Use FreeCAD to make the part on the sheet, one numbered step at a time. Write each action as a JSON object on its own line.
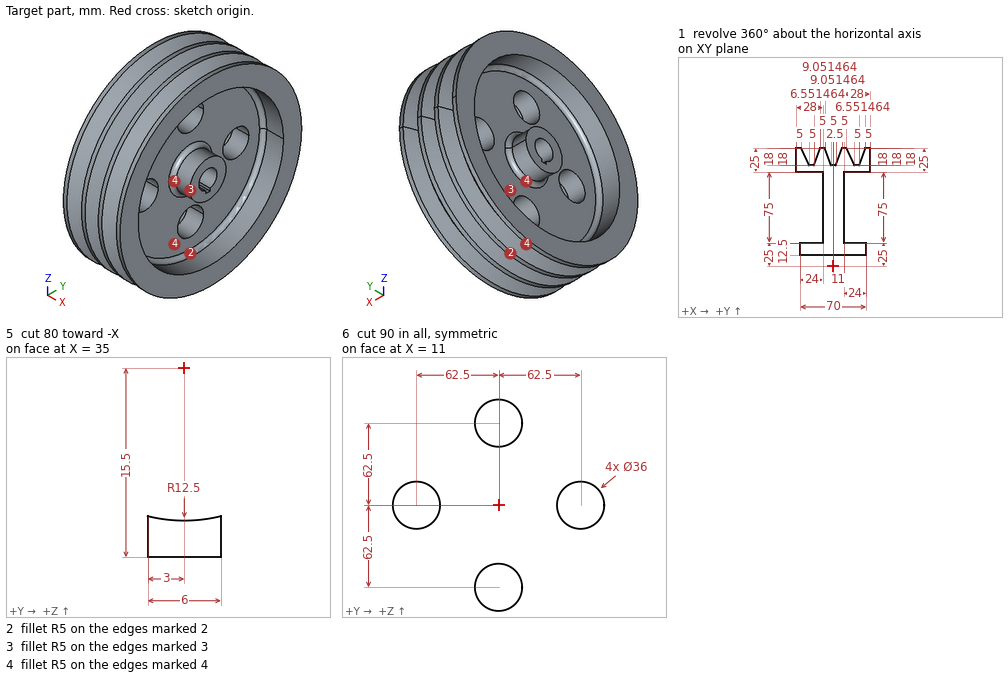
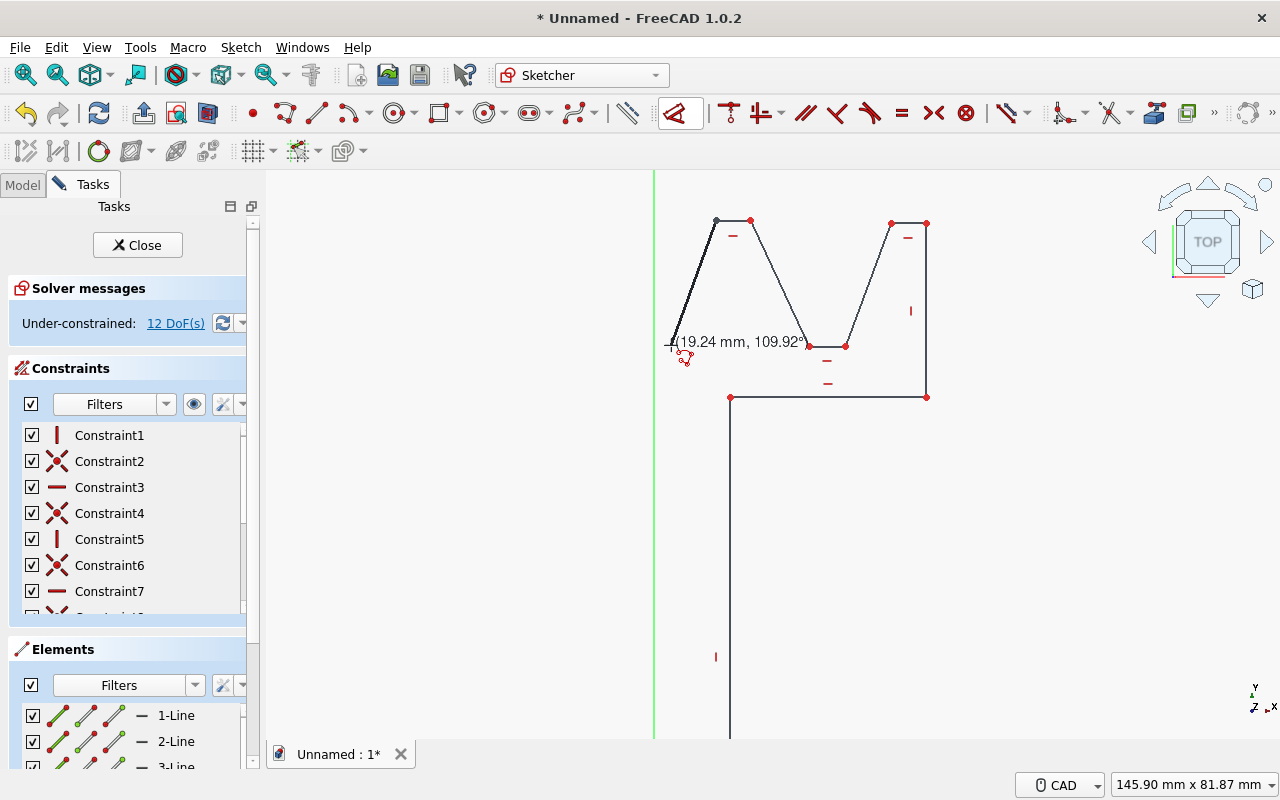
{"action": "left_click", "coordinate": [671, 345]}
{"action": "left_click", "coordinate": [637, 345]}
{"action": "left_click", "coordinate": [591, 220]}
{"action": "left_click", "coordinate": [556, 220]}
{"action": "left_click", "coordinate": [511, 345]}
{"action": "left_click", "coordinate": [476, 345]}
{"action": "left_click", "coordinate": [418, 220]}
{"action": "left_click", "coordinate": [383, 220]}
{"action": "left_click", "coordinate": [383, 394]}
{"action": "left_click", "coordinate": [578, 394]}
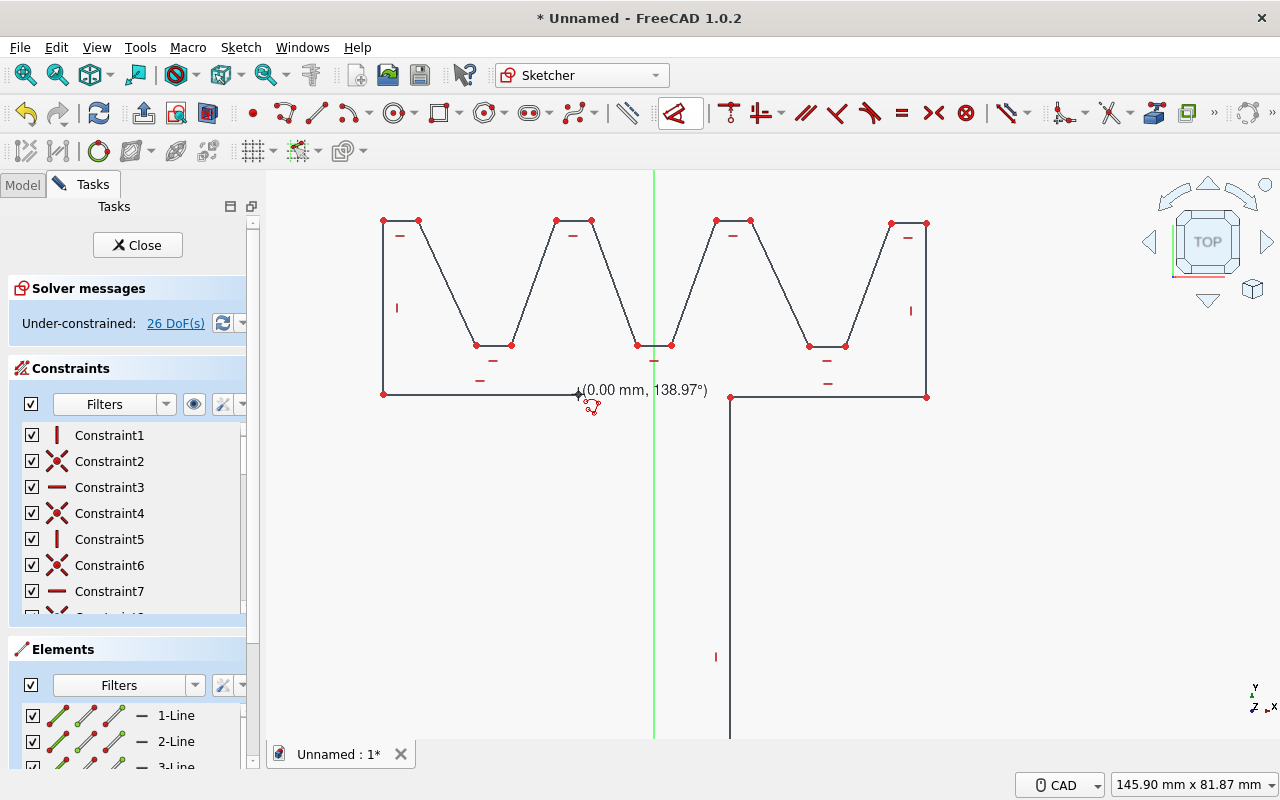
{"action": "scroll", "coordinate": [746, 292], "scroll_direction": "down", "scroll_amount": 4}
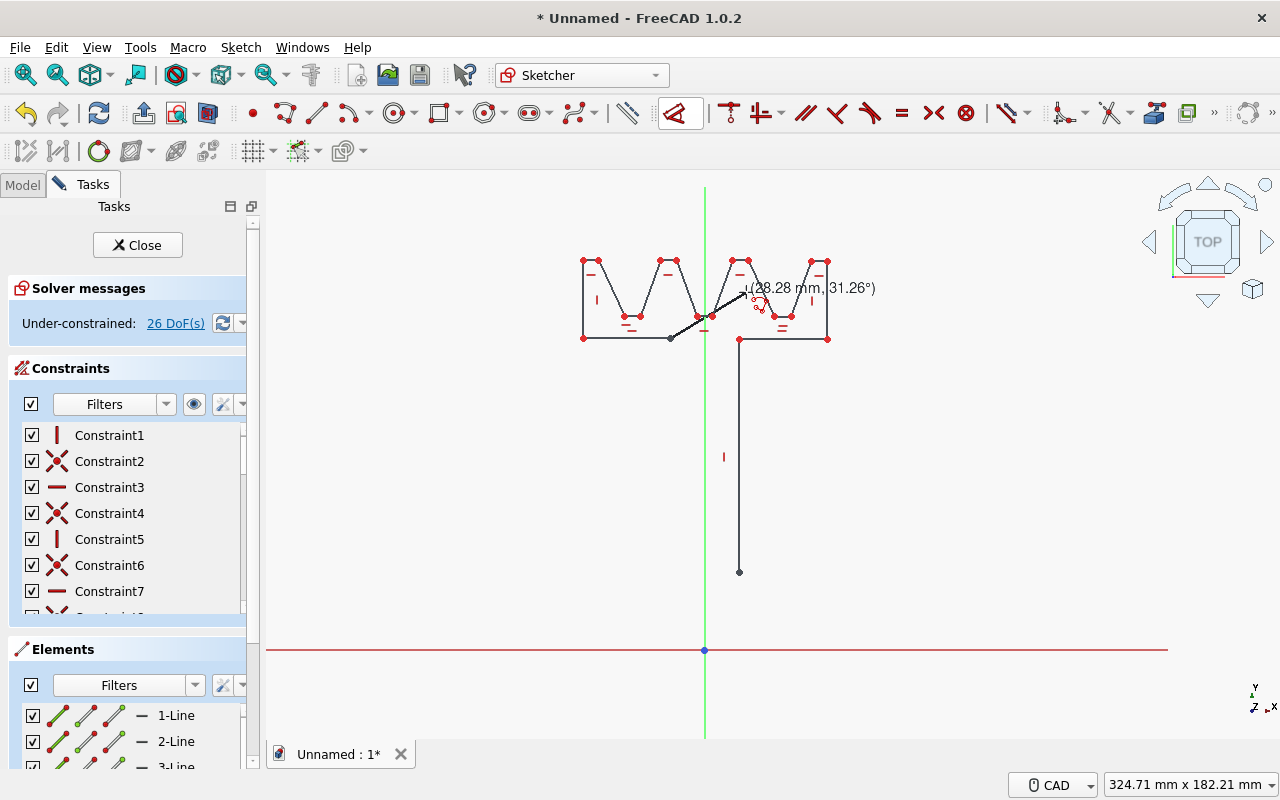
{"action": "left_click", "coordinate": [671, 572]}
{"action": "left_click", "coordinate": [596, 572]}
{"action": "left_click", "coordinate": [596, 611]}
{"action": "left_click", "coordinate": [814, 611]}
{"action": "left_click", "coordinate": [814, 572]}
{"action": "left_click", "coordinate": [739, 573]}
{"action": "key", "text": "Escape"}
{"action": "key", "text": "Escape"}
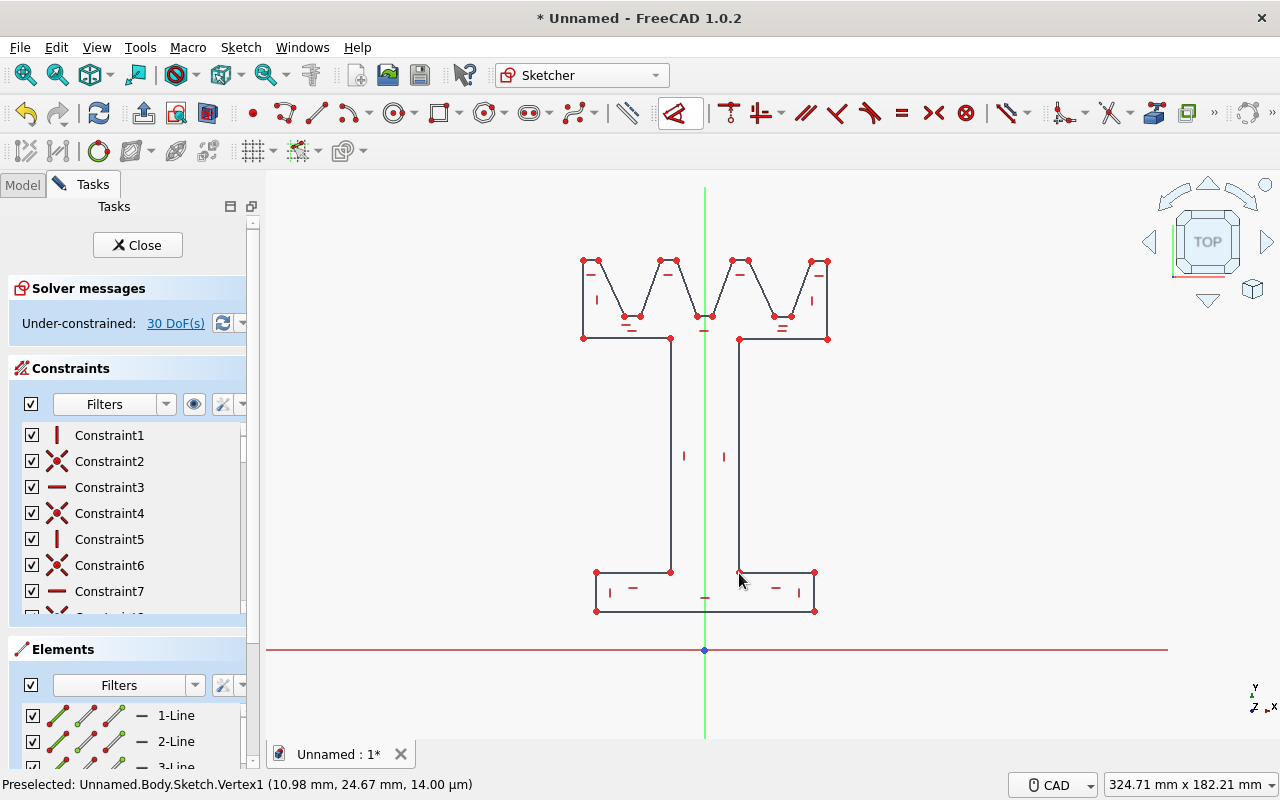
{"action": "scroll", "coordinate": [819, 261], "scroll_direction": "up", "scroll_amount": 5}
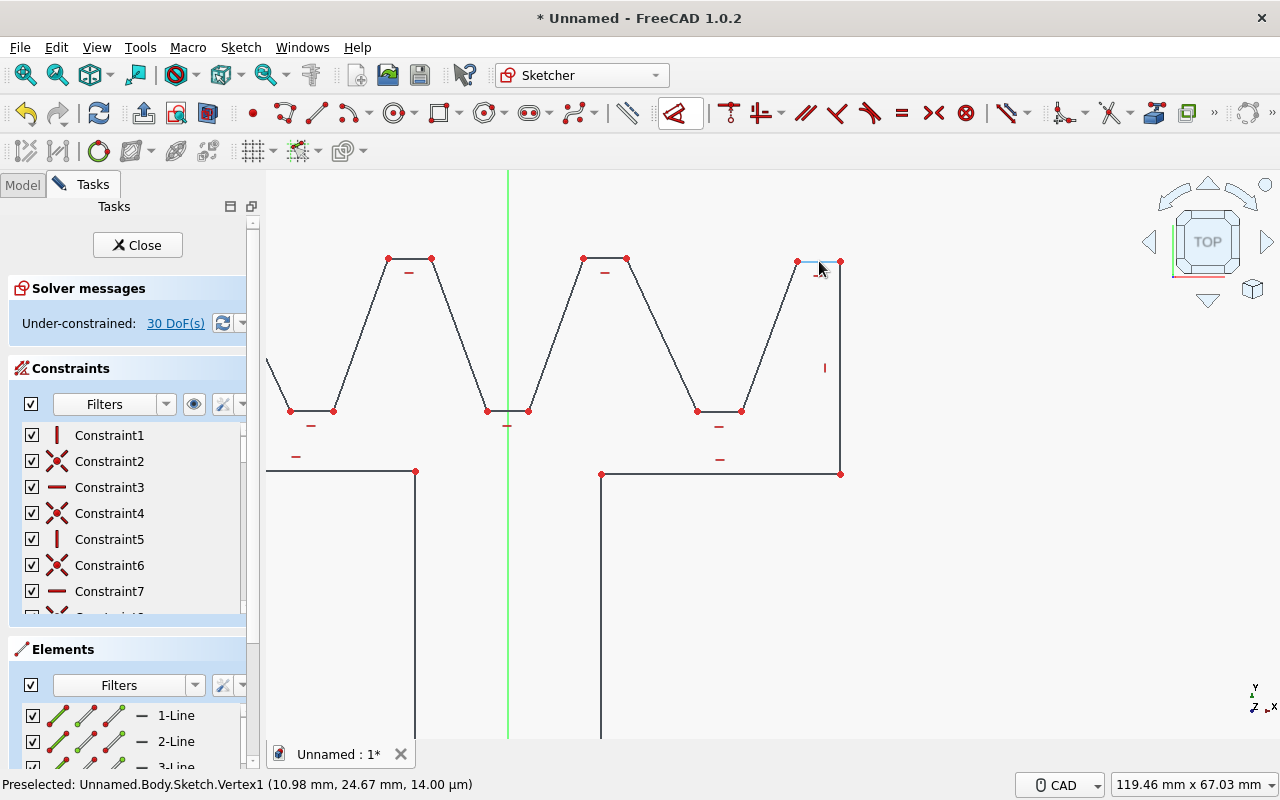
{"action": "left_click", "coordinate": [819, 262]}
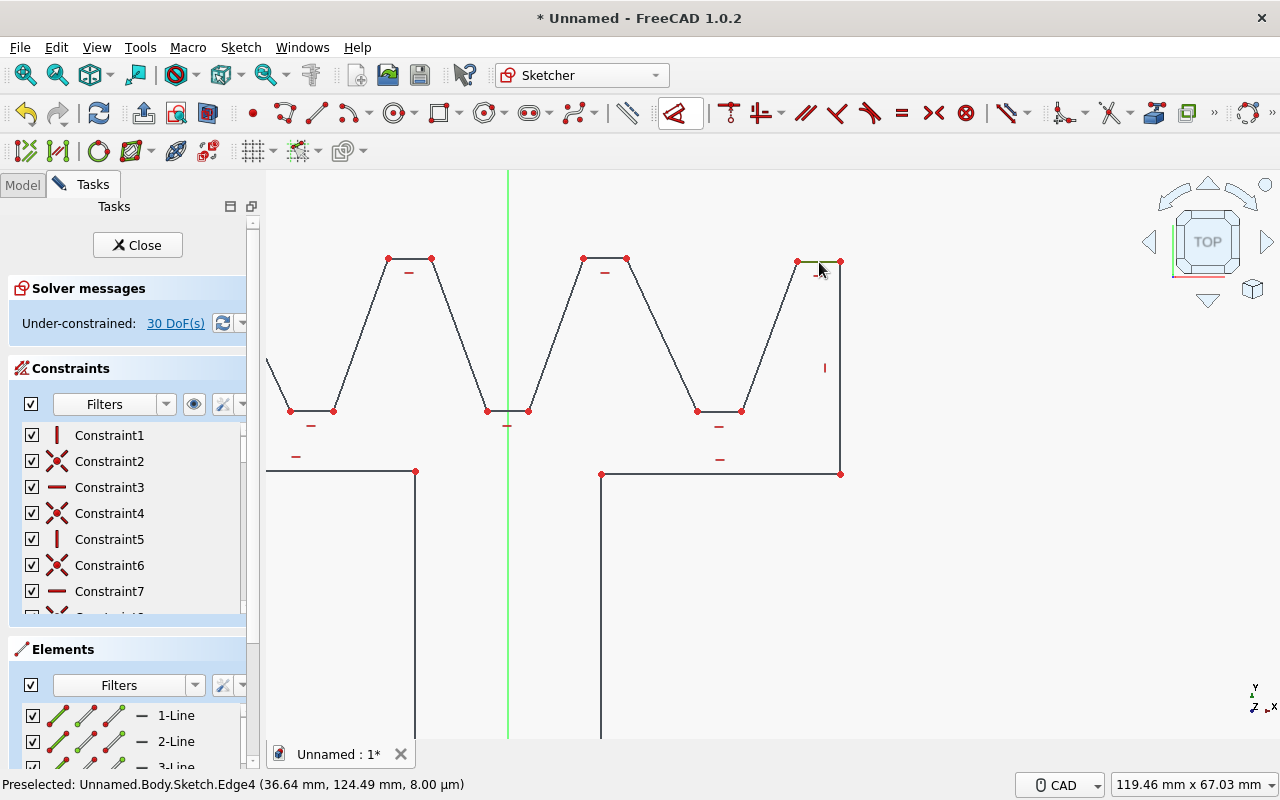
{"action": "left_click", "coordinate": [698, 114]}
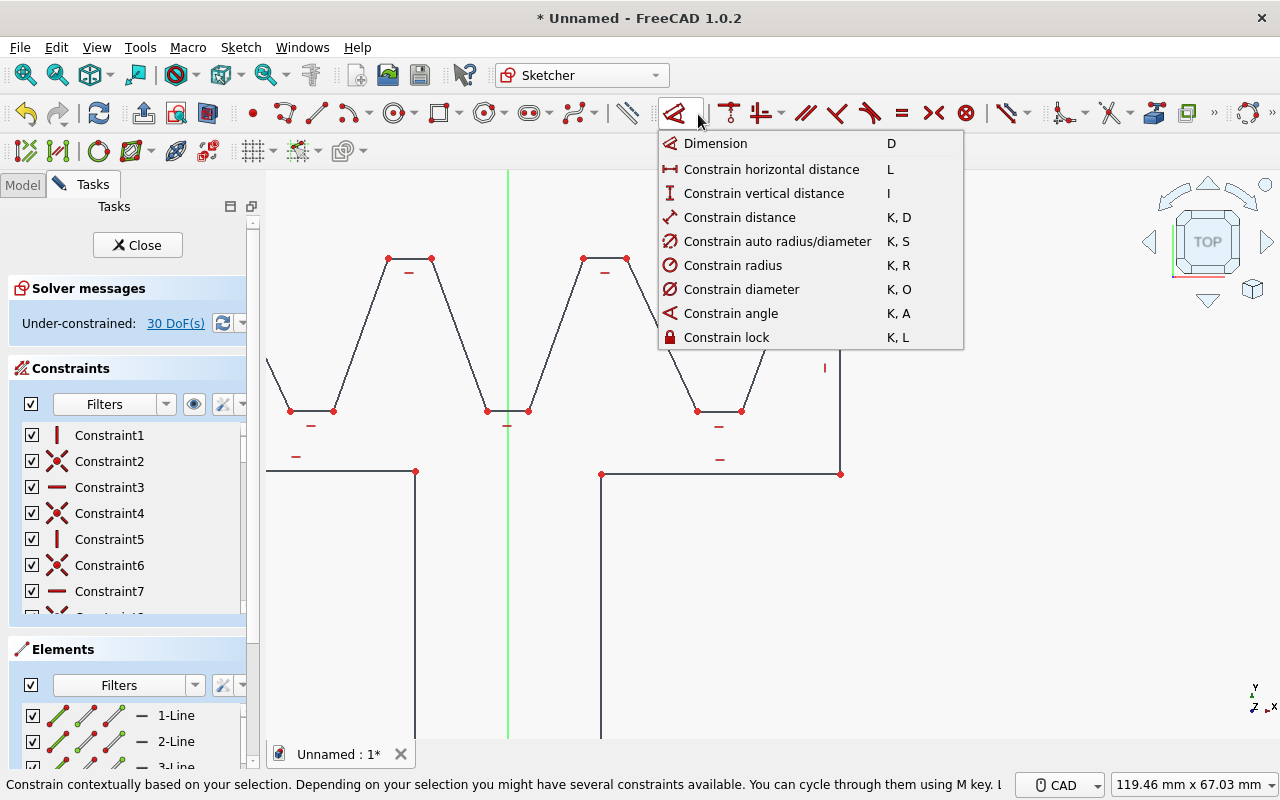
{"action": "left_click", "coordinate": [811, 169]}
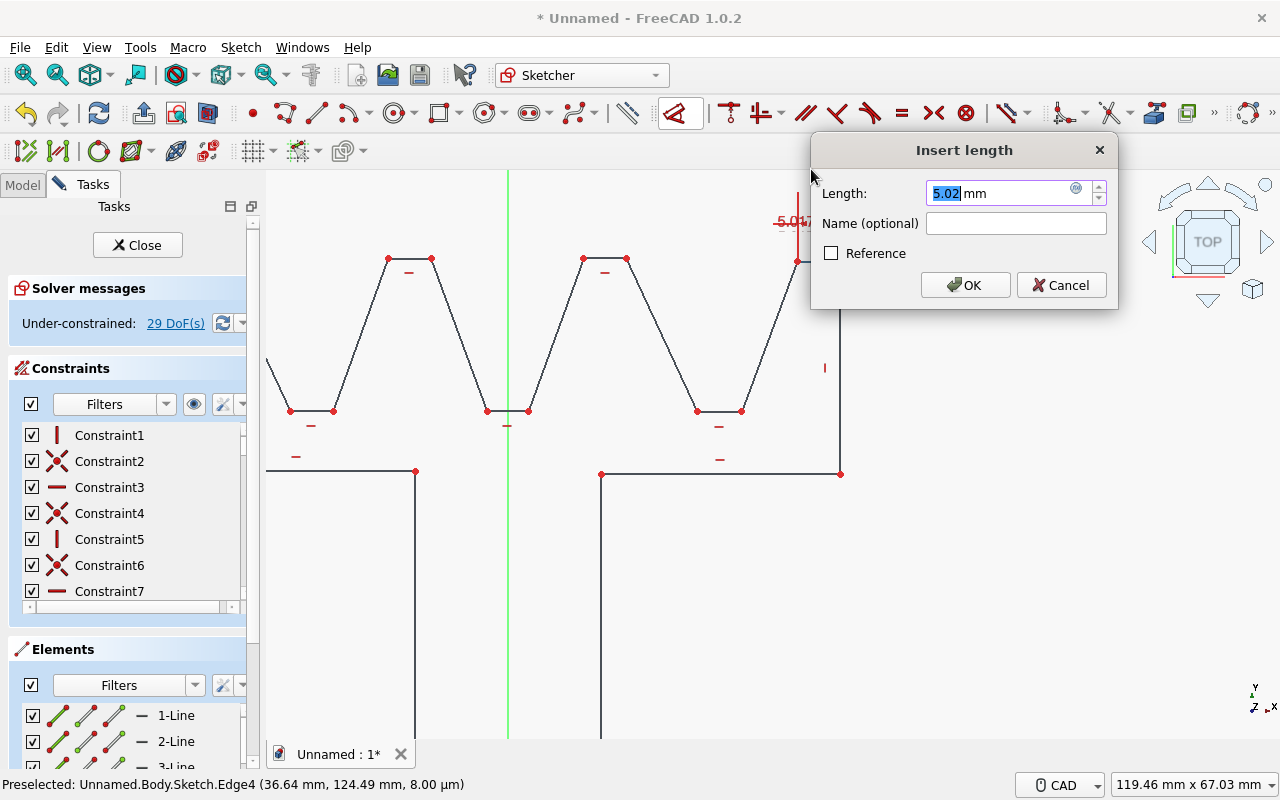
{"action": "type", "text": "5"}
{"action": "key", "text": "Return"}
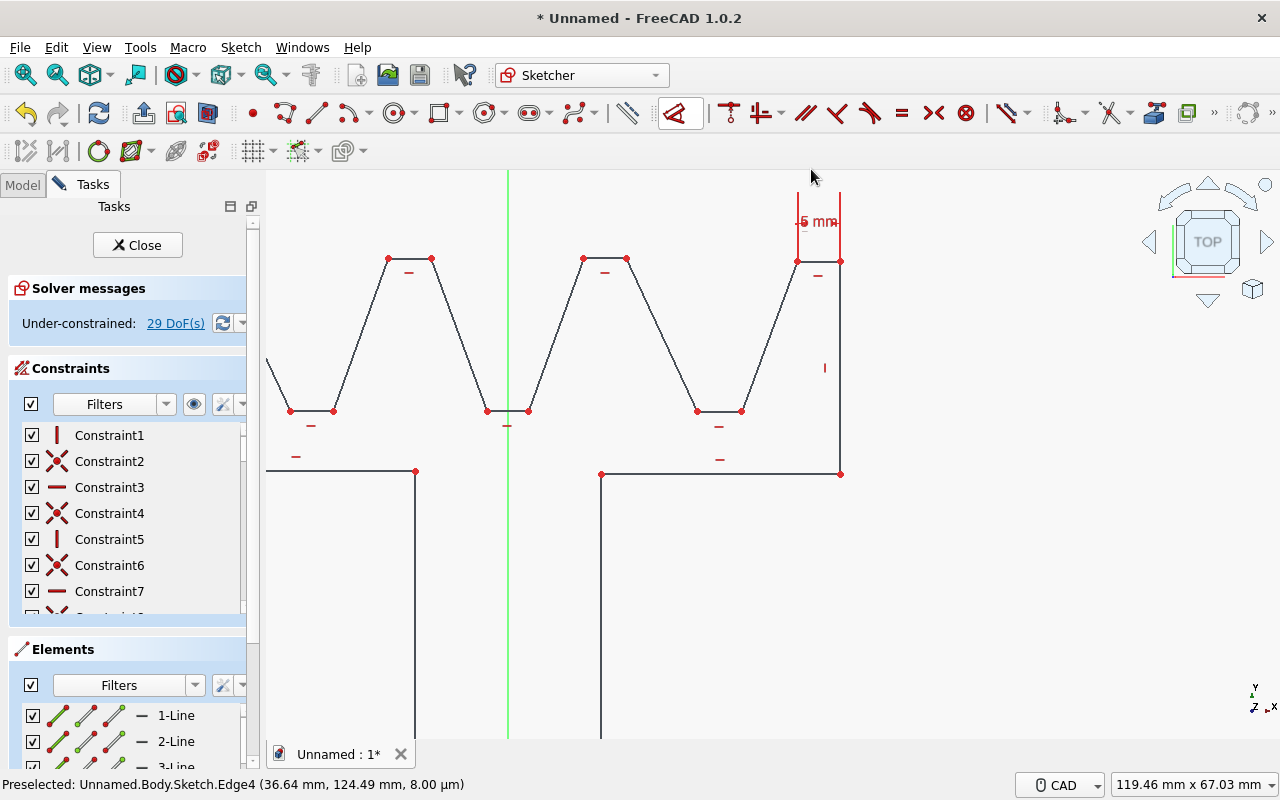
{"action": "left_click", "coordinate": [729, 412]}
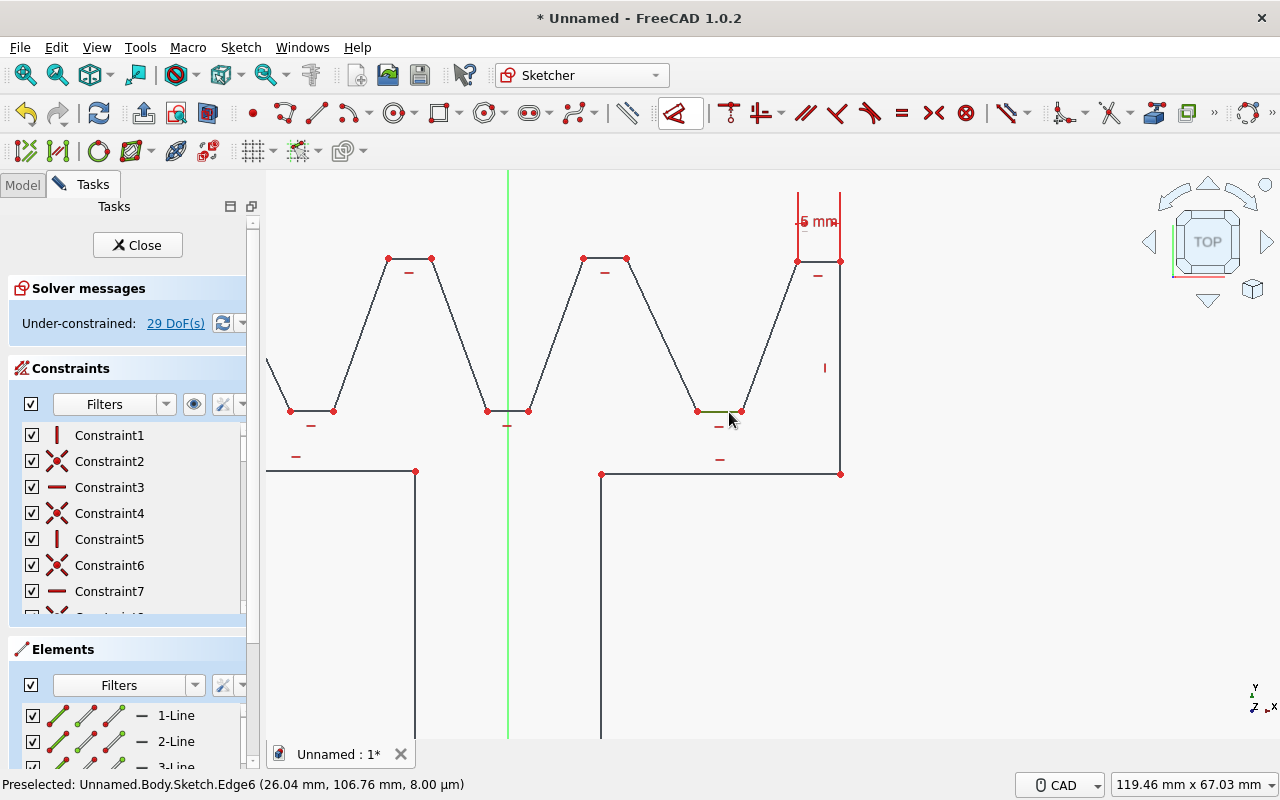
{"action": "key", "text": "l"}